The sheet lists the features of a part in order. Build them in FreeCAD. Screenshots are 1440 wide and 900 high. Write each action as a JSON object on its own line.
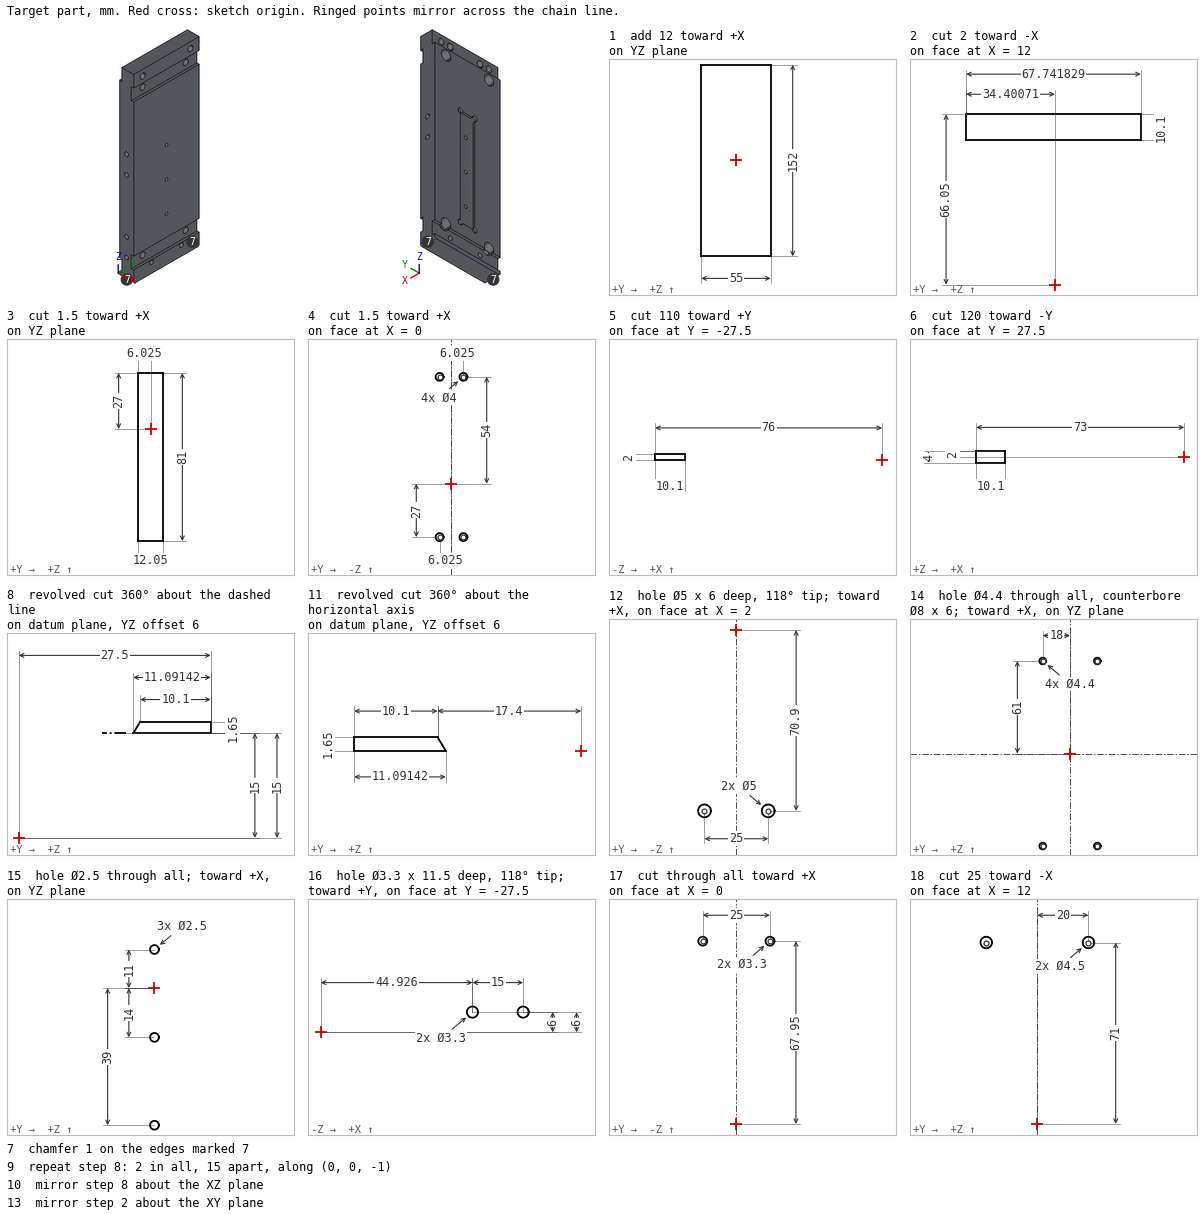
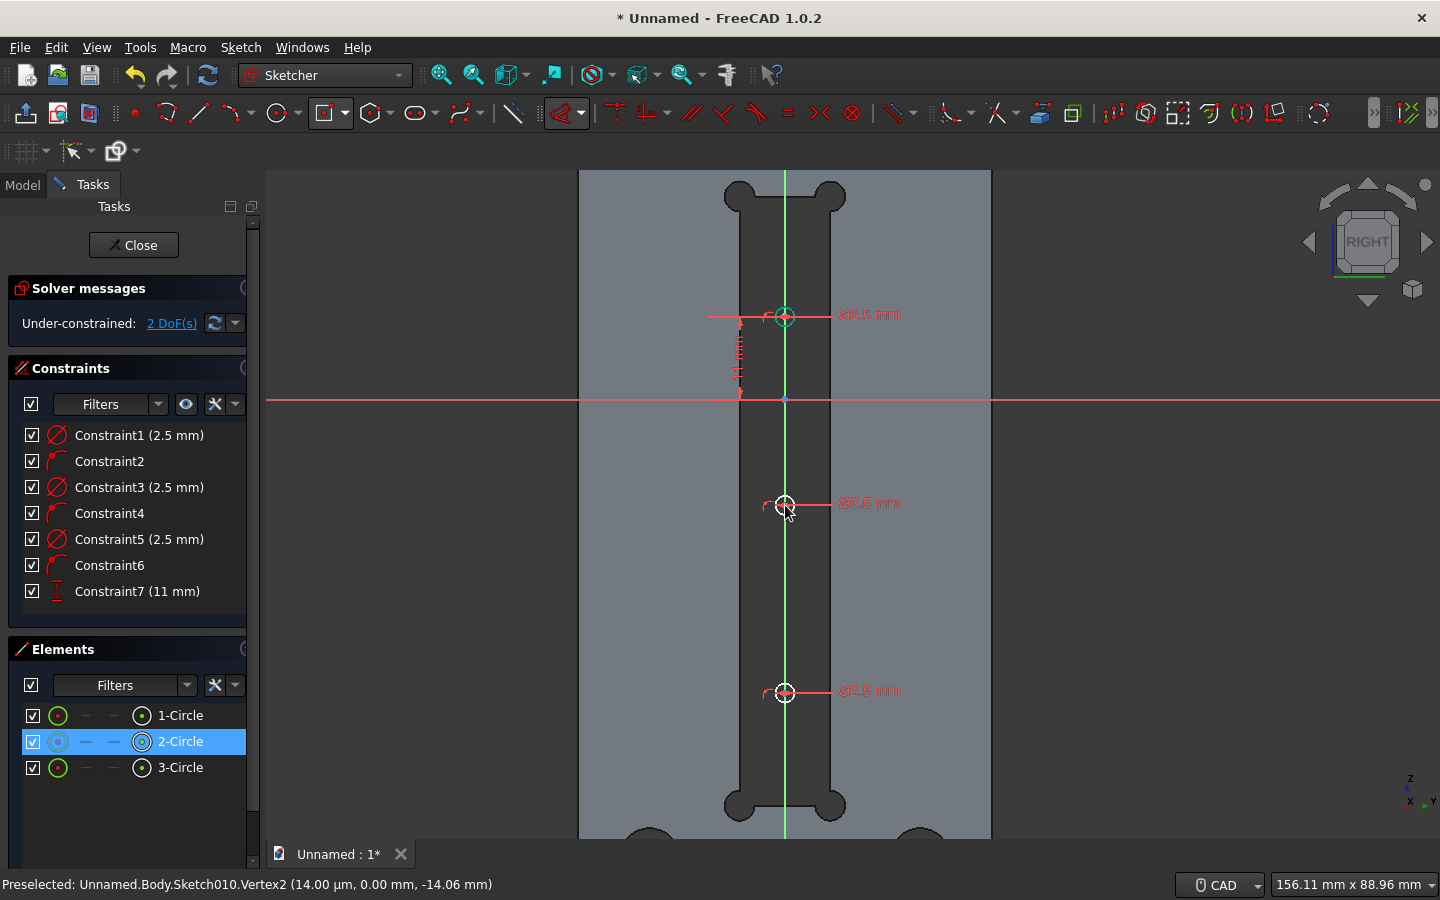
{"action": "left_click", "coordinate": [584, 114]}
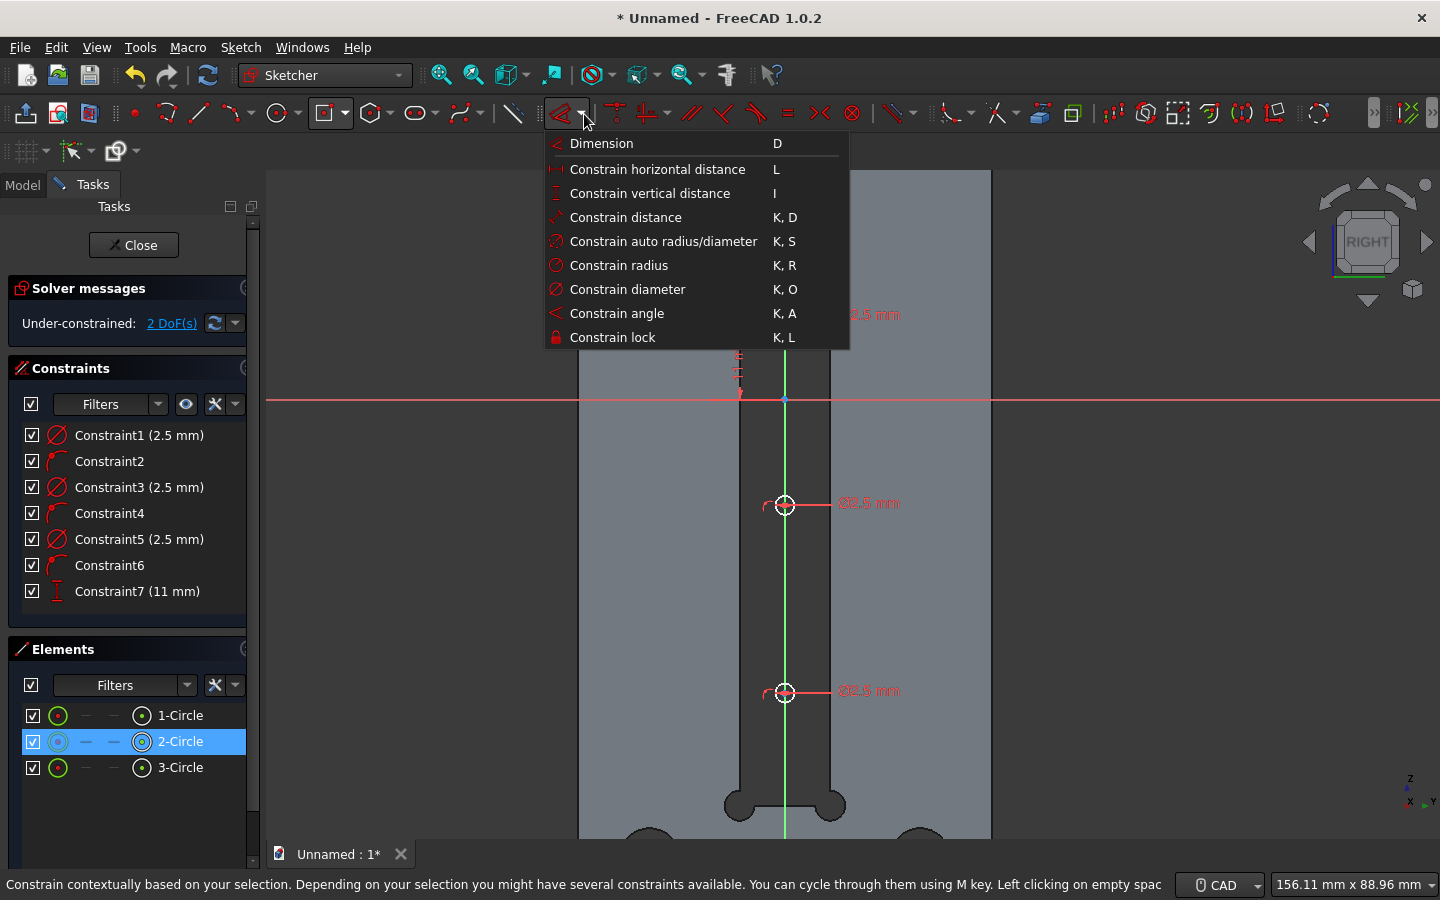
{"action": "left_click", "coordinate": [697, 193]}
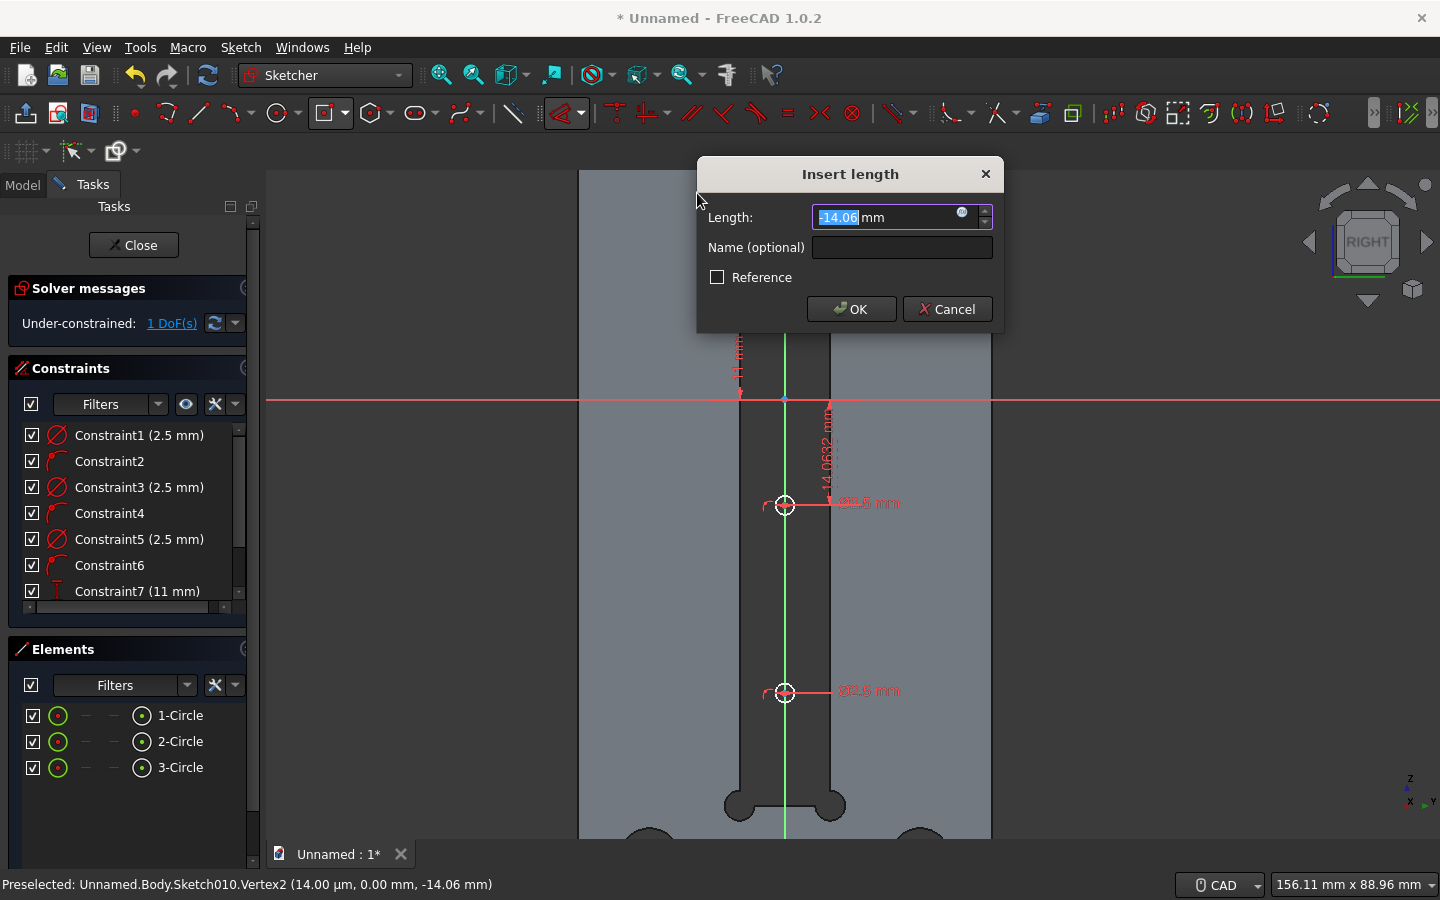
{"action": "type", "text": "-14"}
{"action": "key", "text": "Return"}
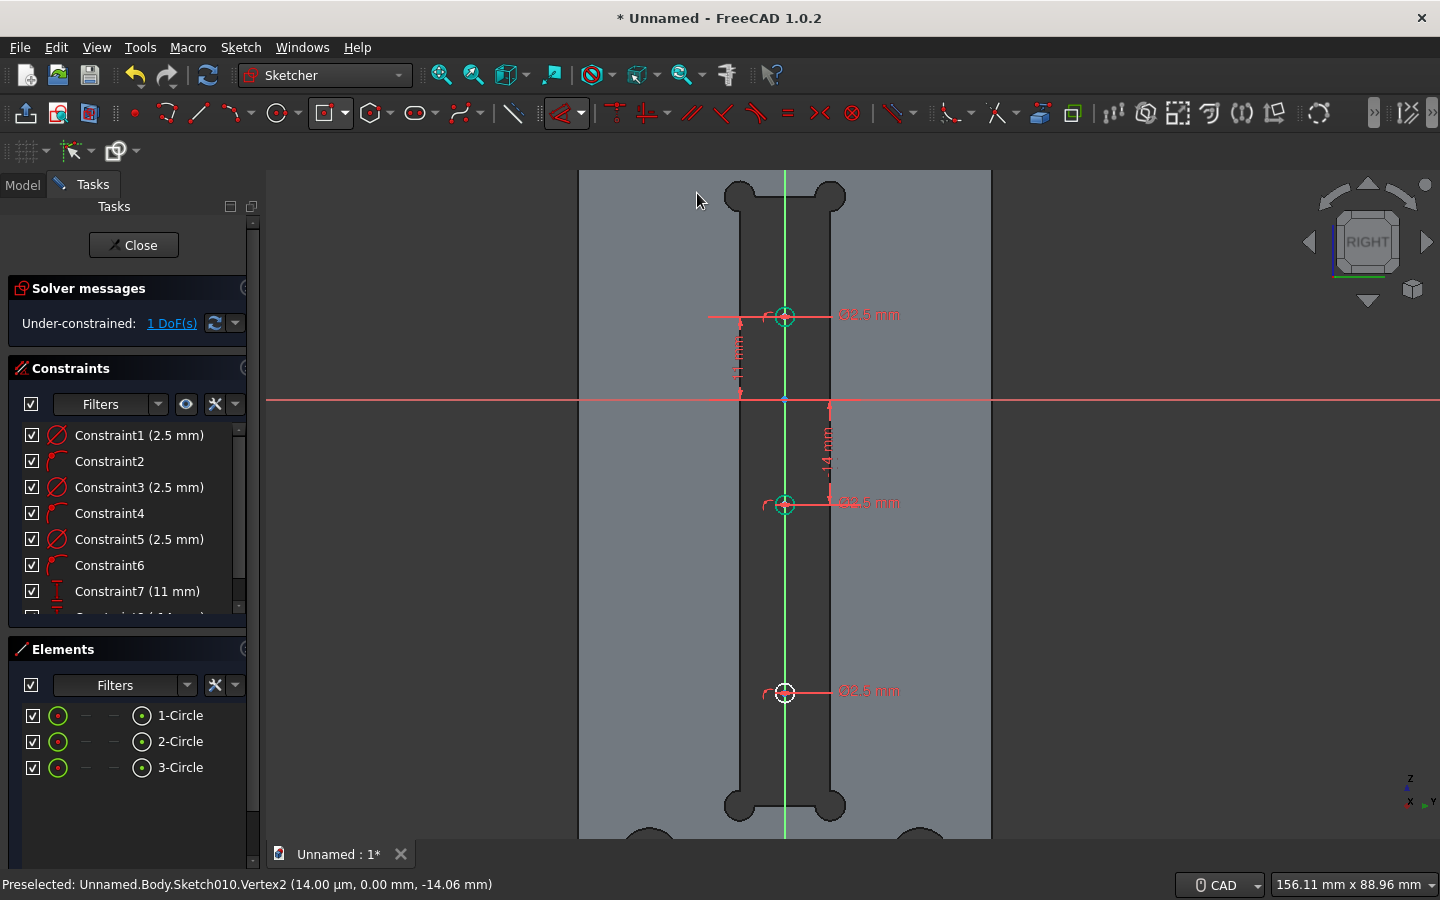
{"action": "left_click", "coordinate": [785, 693]}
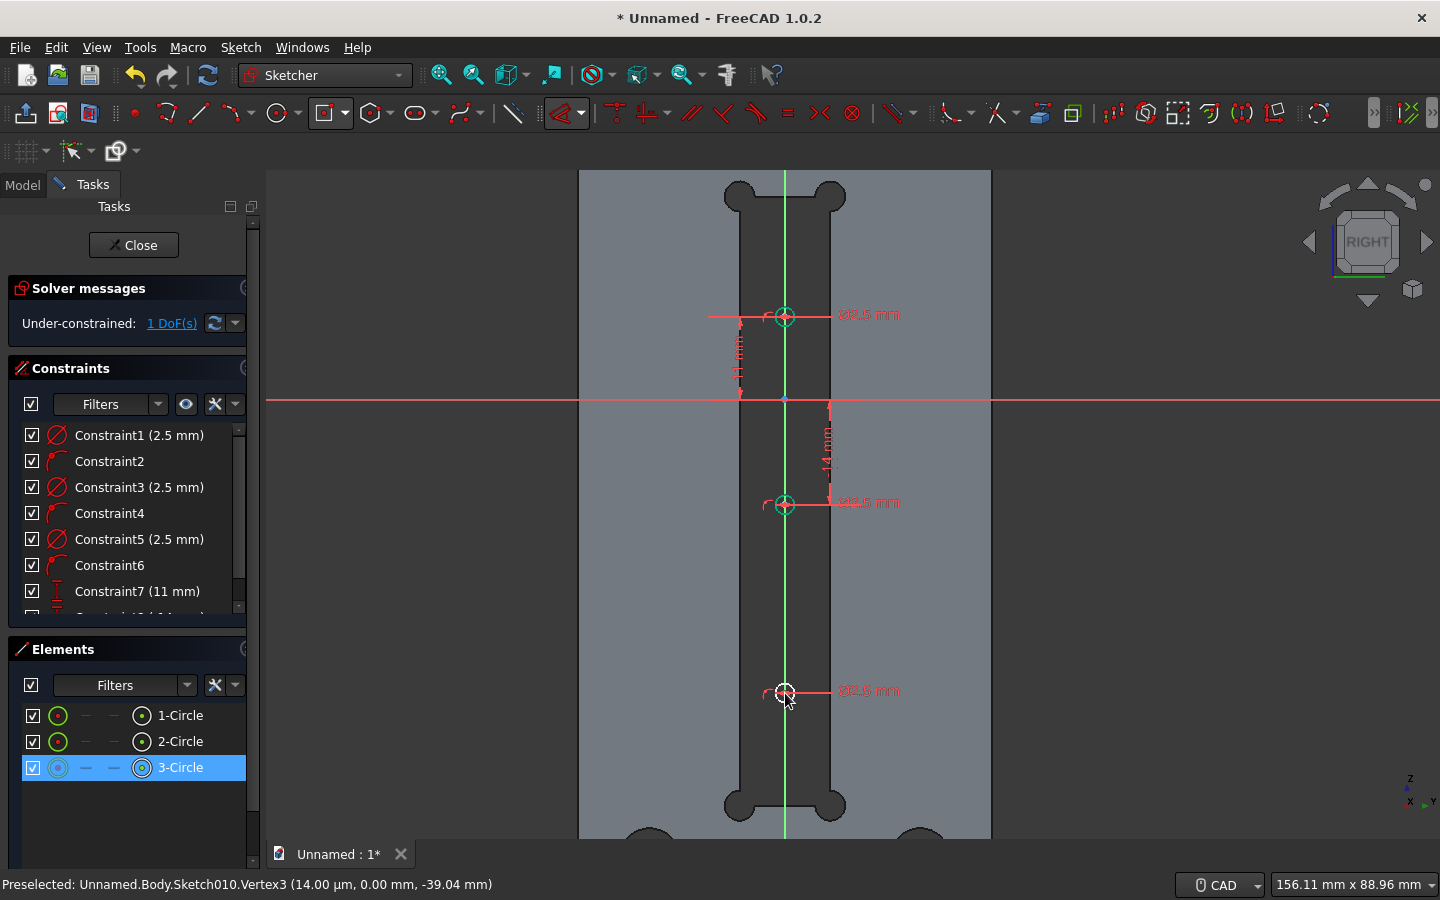
{"action": "left_click", "coordinate": [584, 114]}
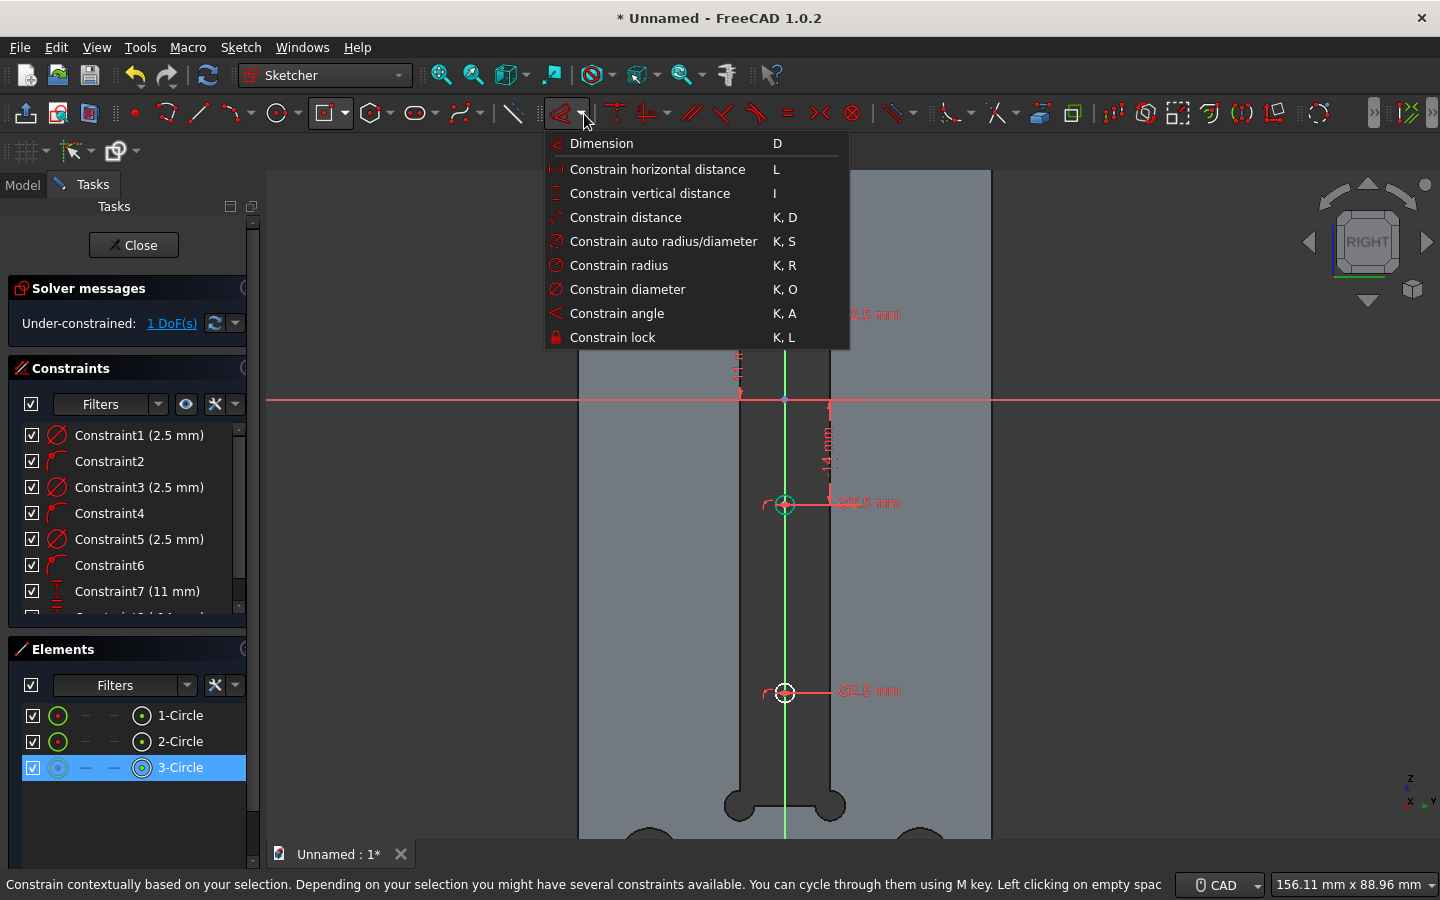
{"action": "left_click", "coordinate": [697, 193]}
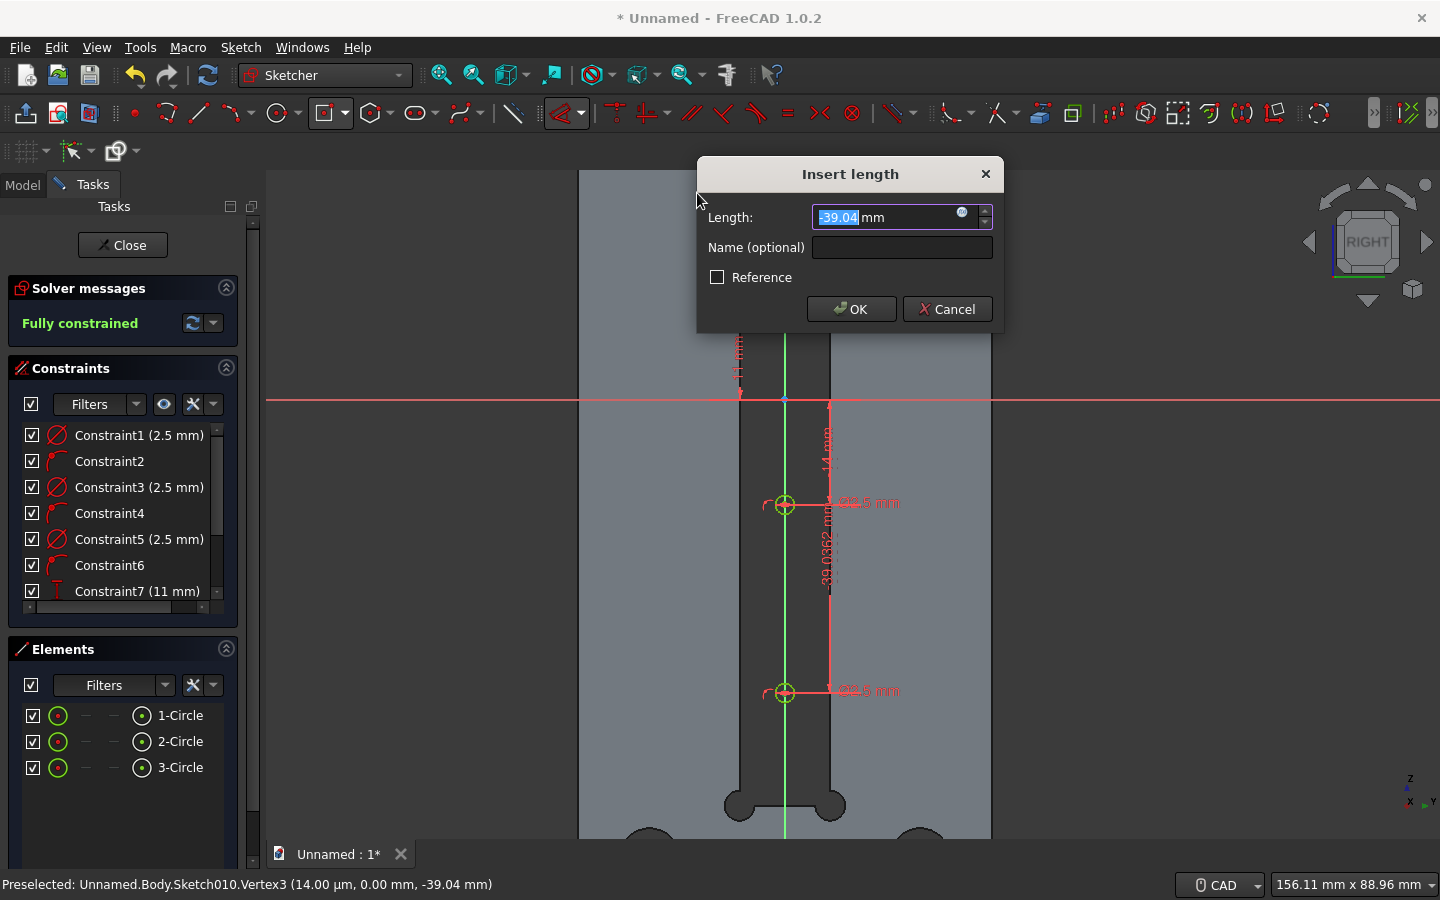
{"action": "type", "text": "-39"}
{"action": "key", "text": "Return"}